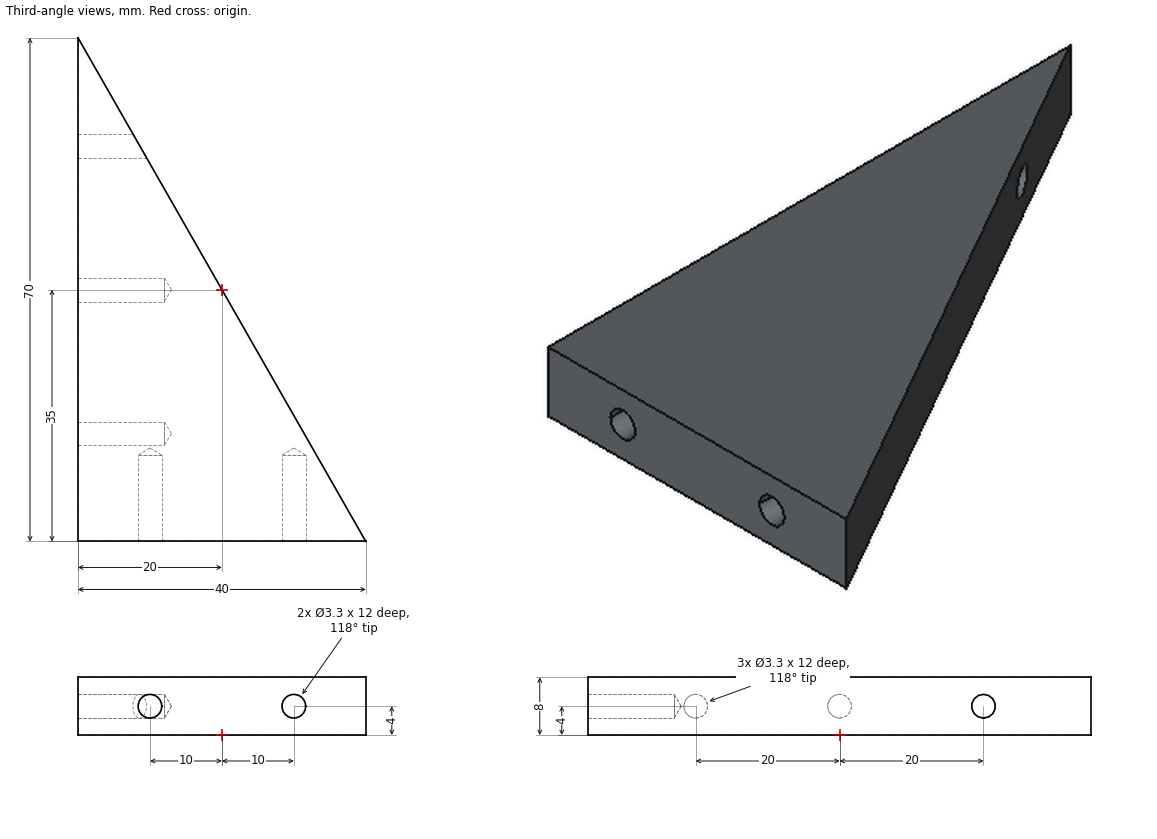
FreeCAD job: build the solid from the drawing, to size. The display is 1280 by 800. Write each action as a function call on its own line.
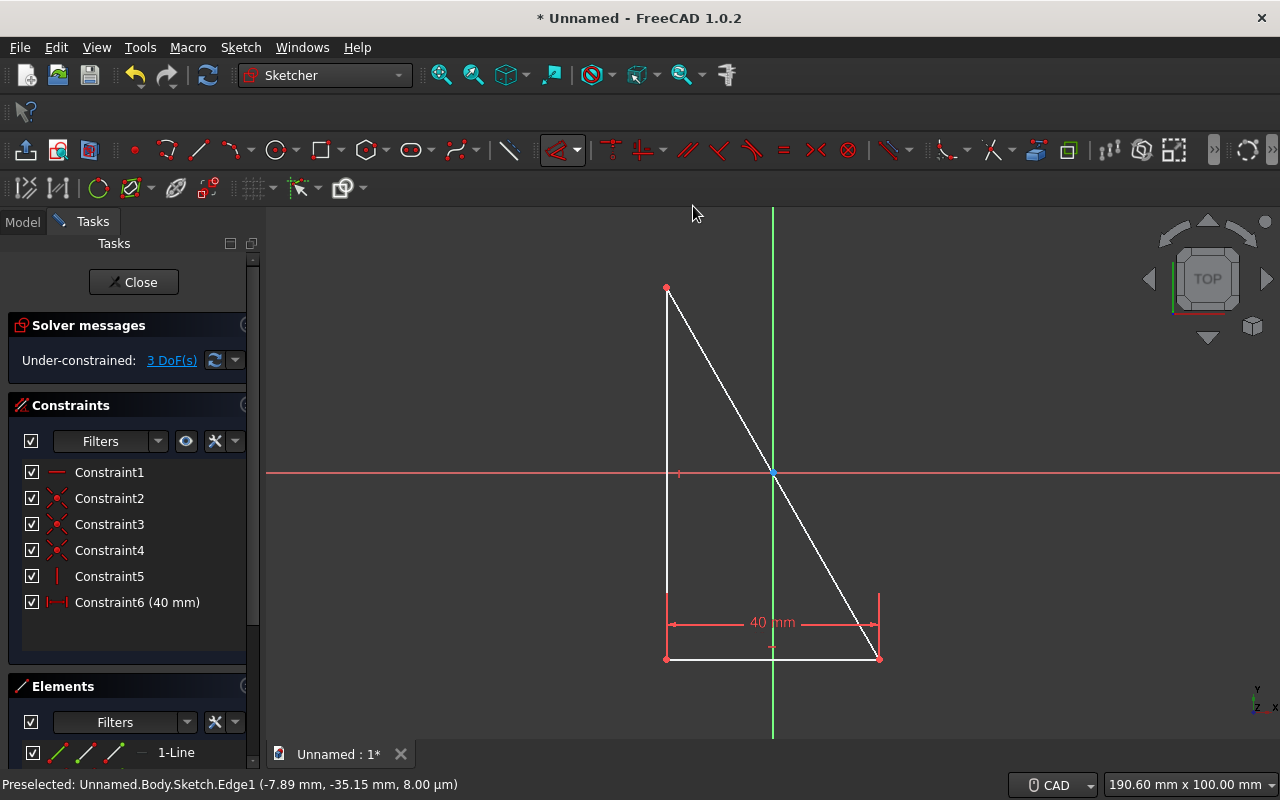
click(667, 400)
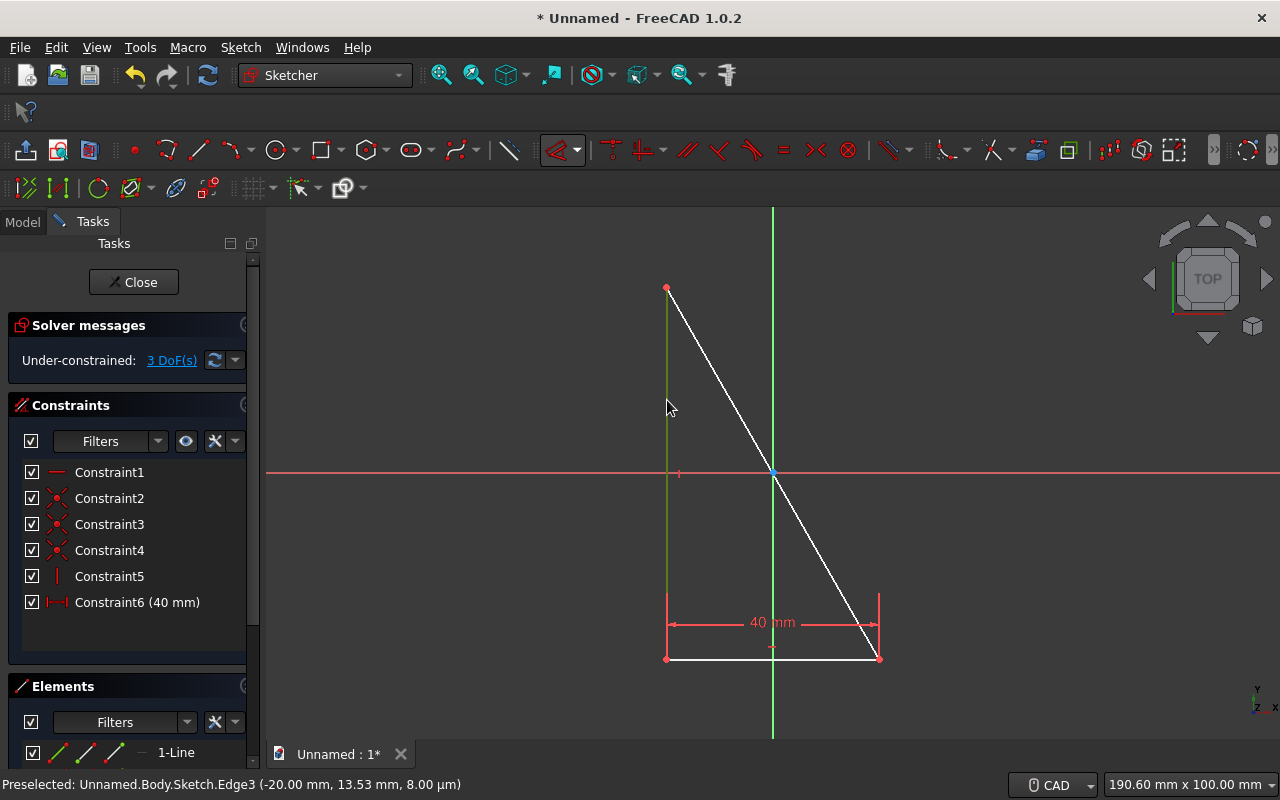
key(i)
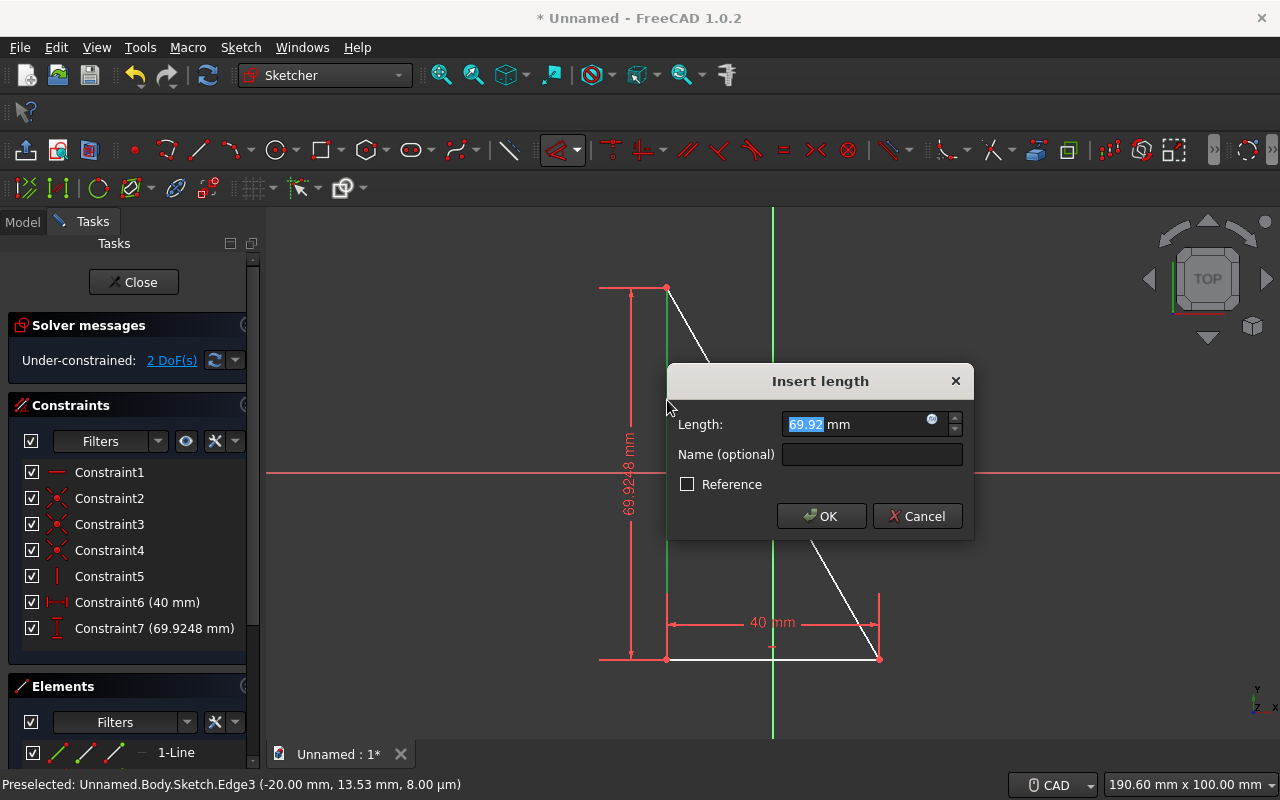
text(70)
key(Return)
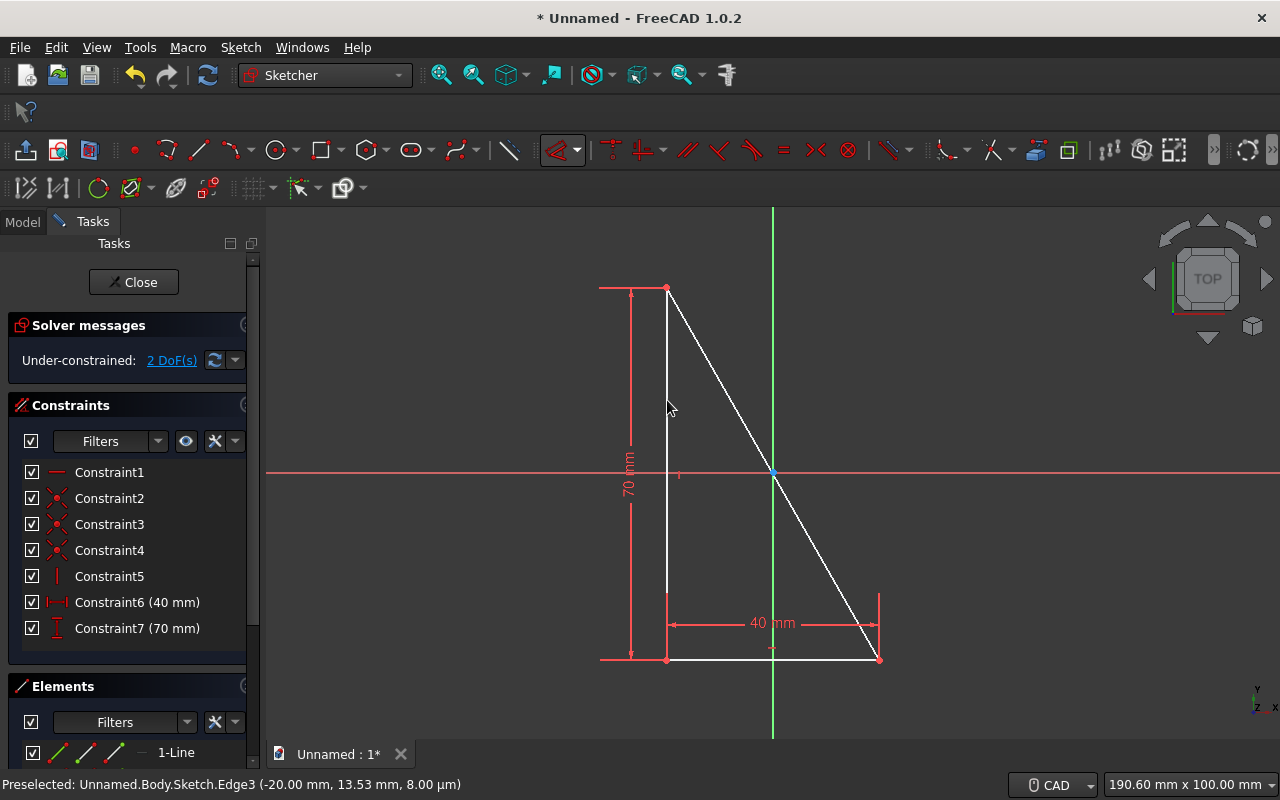
click(667, 660)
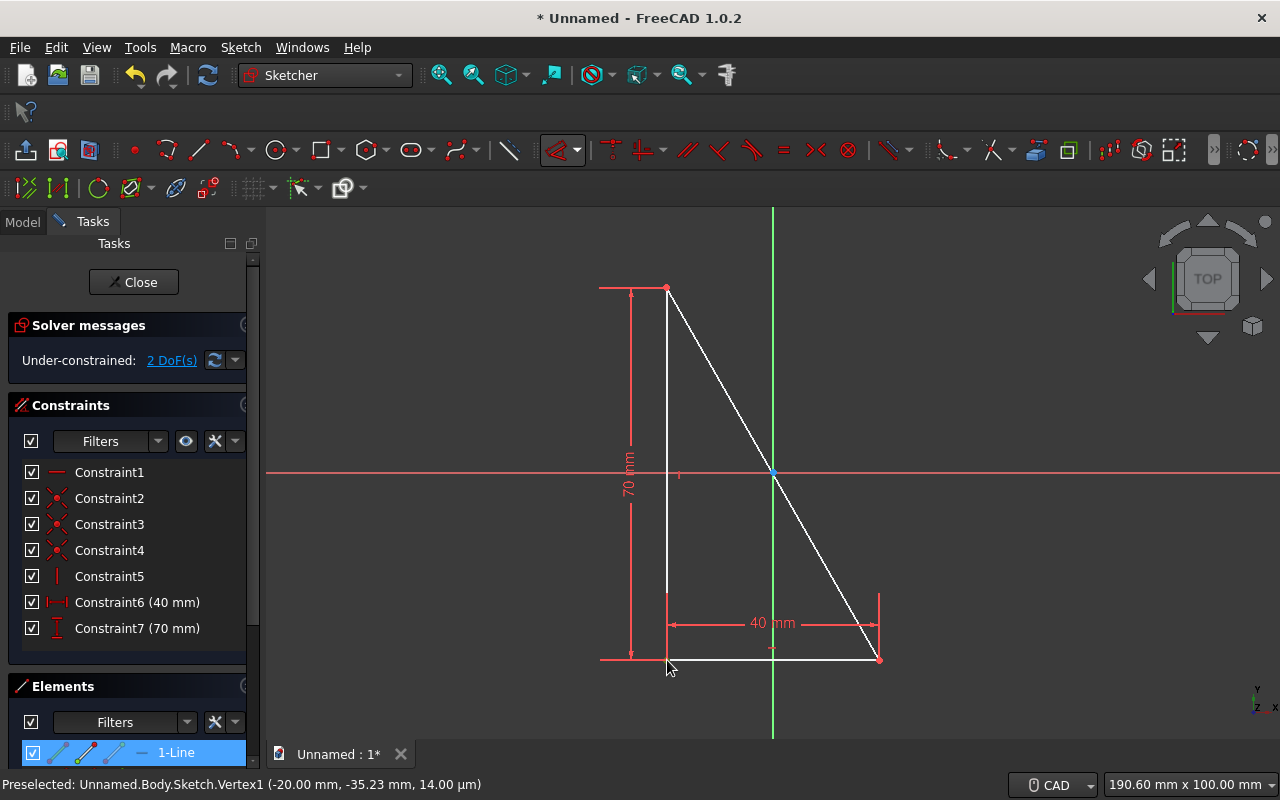
key(l)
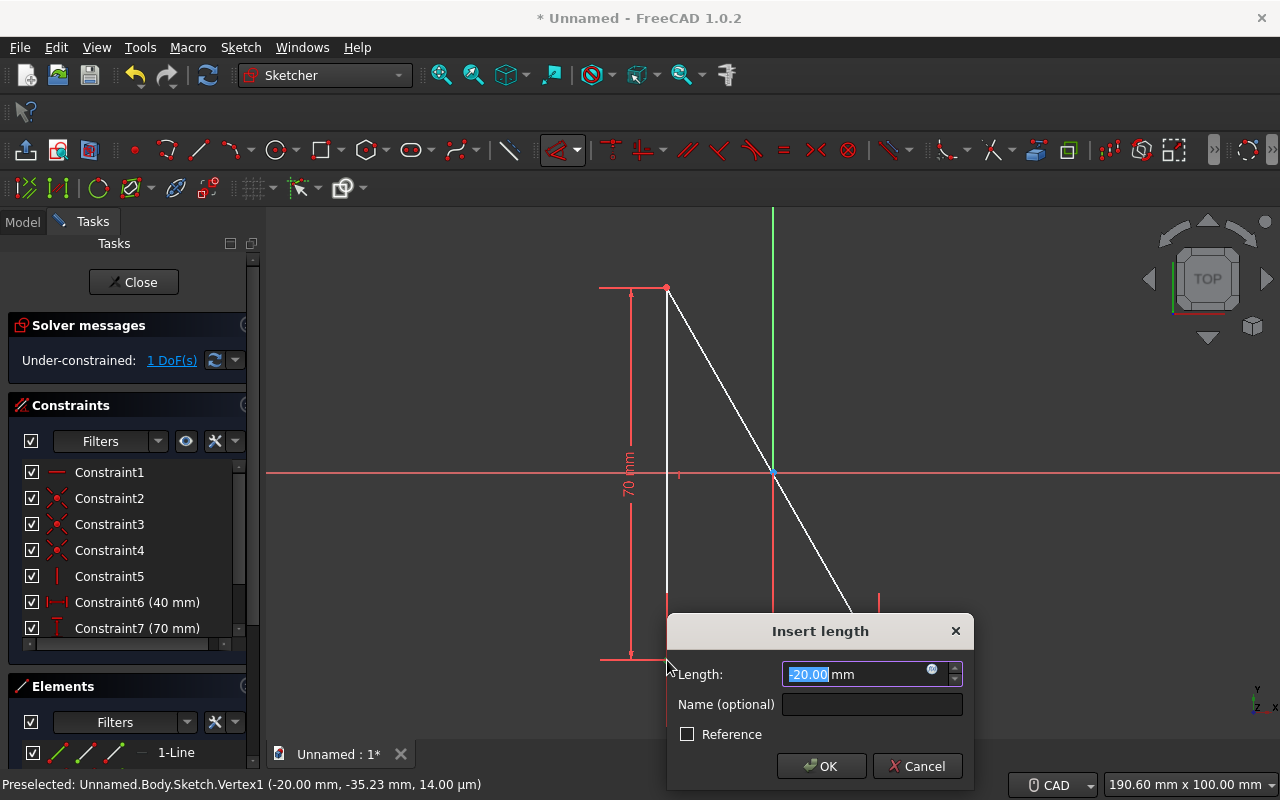
text(-20)
key(Return)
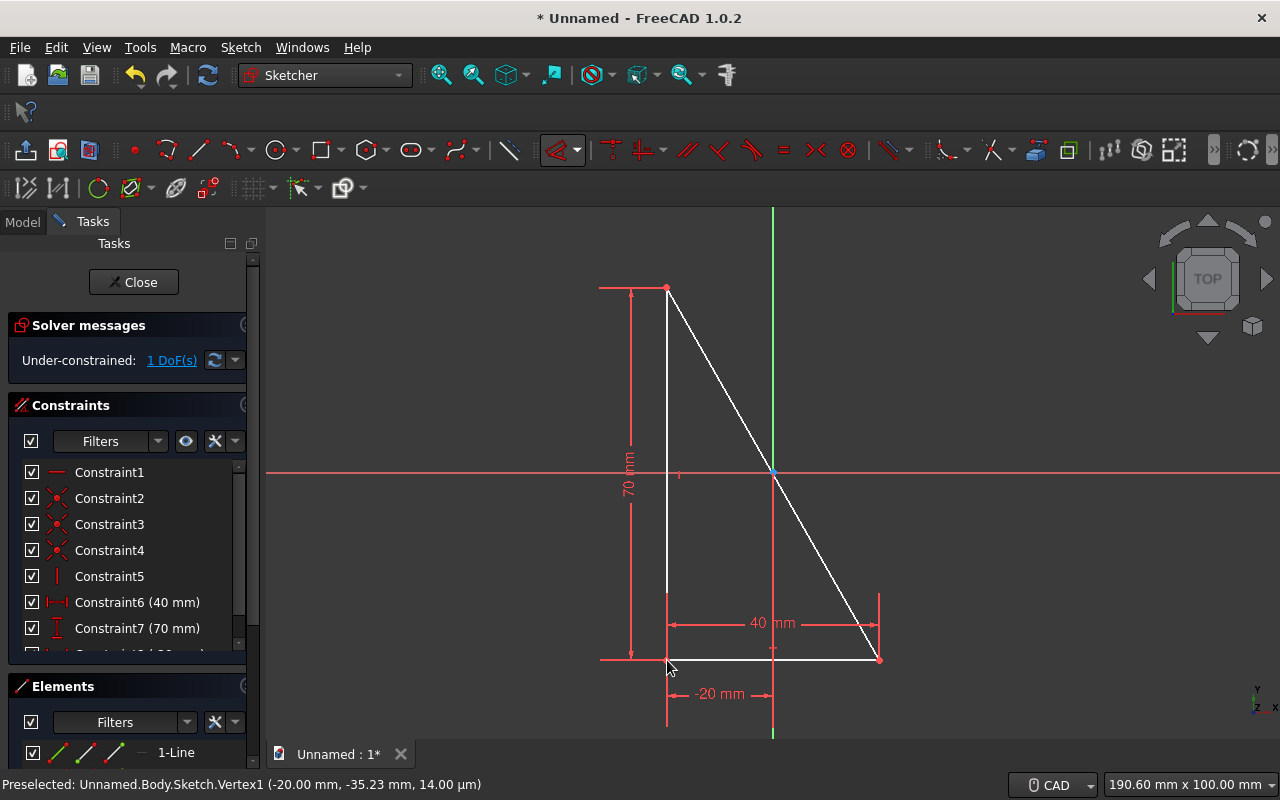
click(667, 660)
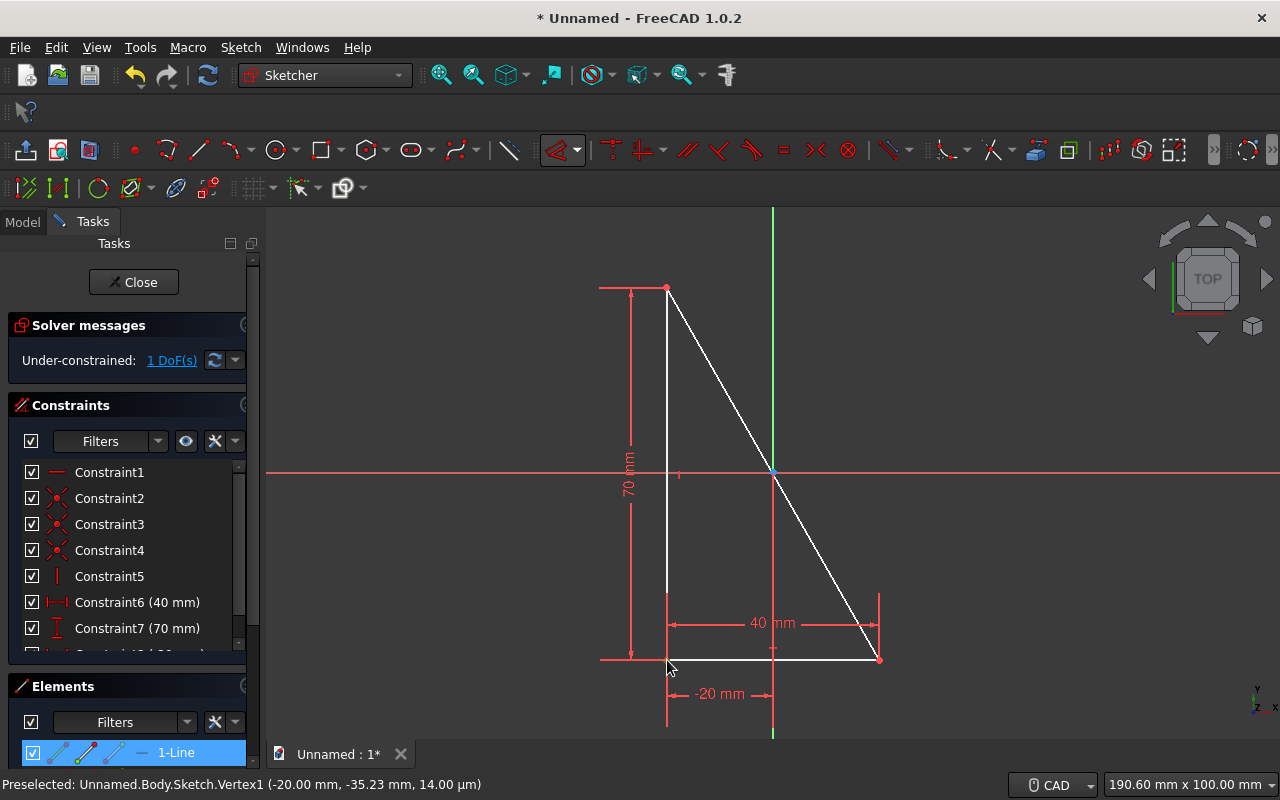
key(i)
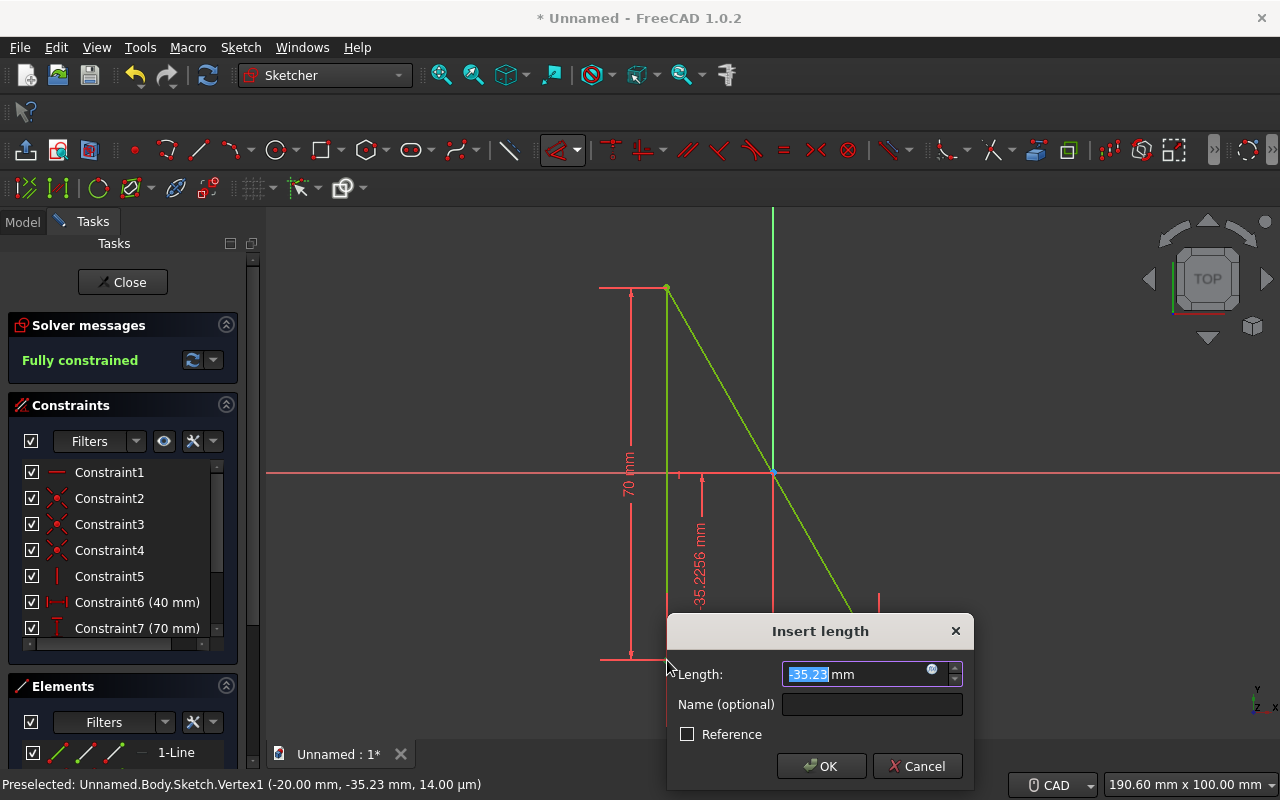
text(-35)
key(Return)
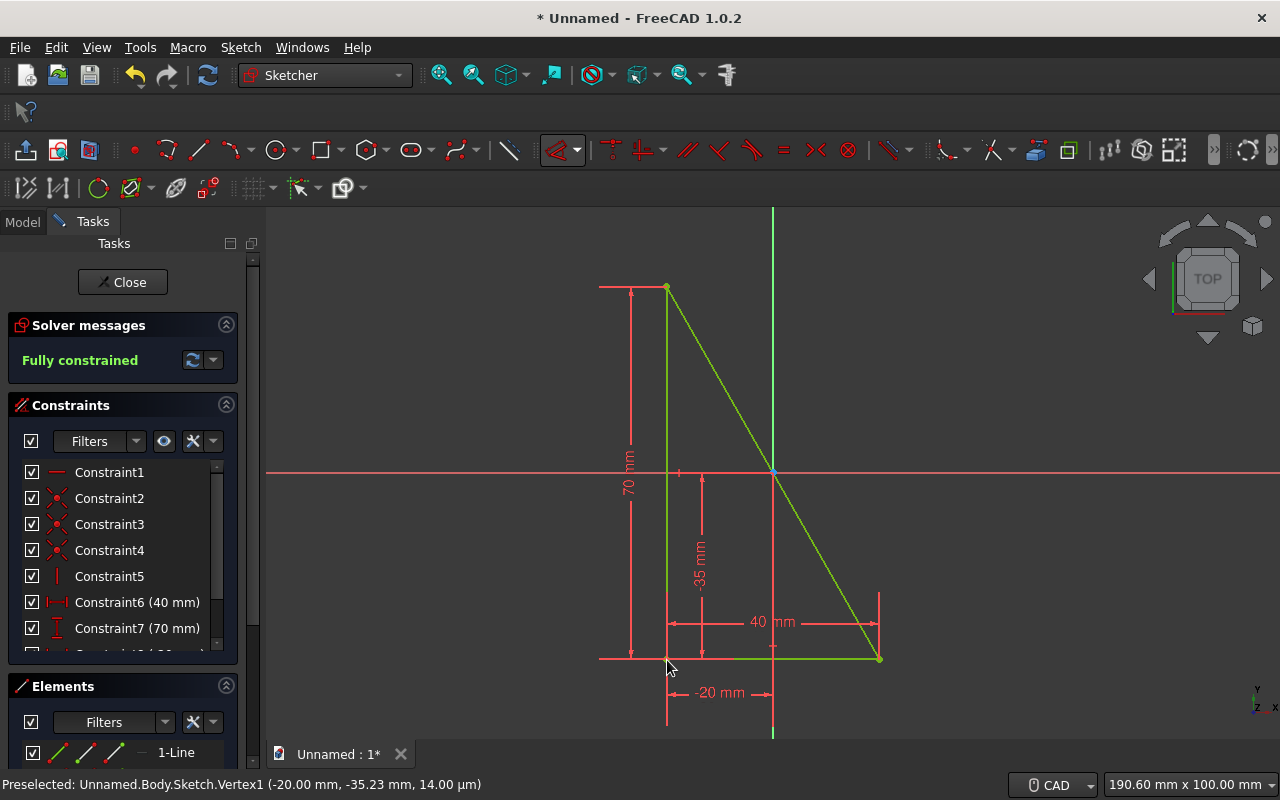
click(123, 282)